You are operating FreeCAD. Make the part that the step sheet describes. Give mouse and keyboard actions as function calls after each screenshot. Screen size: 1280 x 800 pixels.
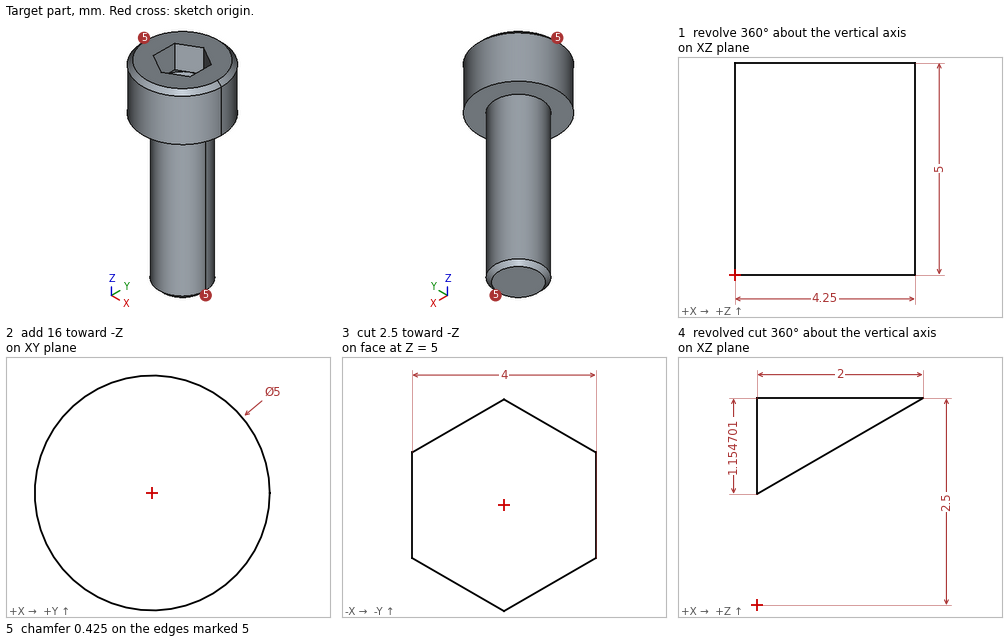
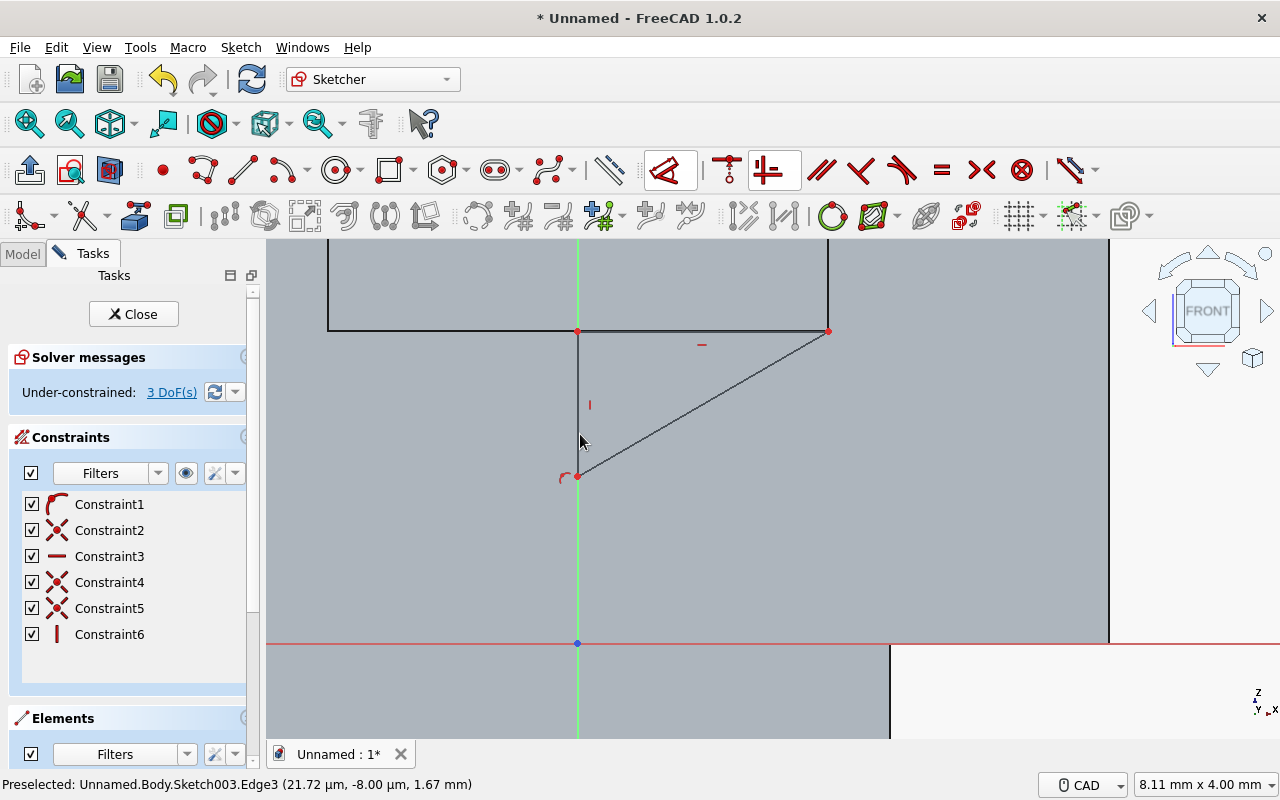
click(753, 332)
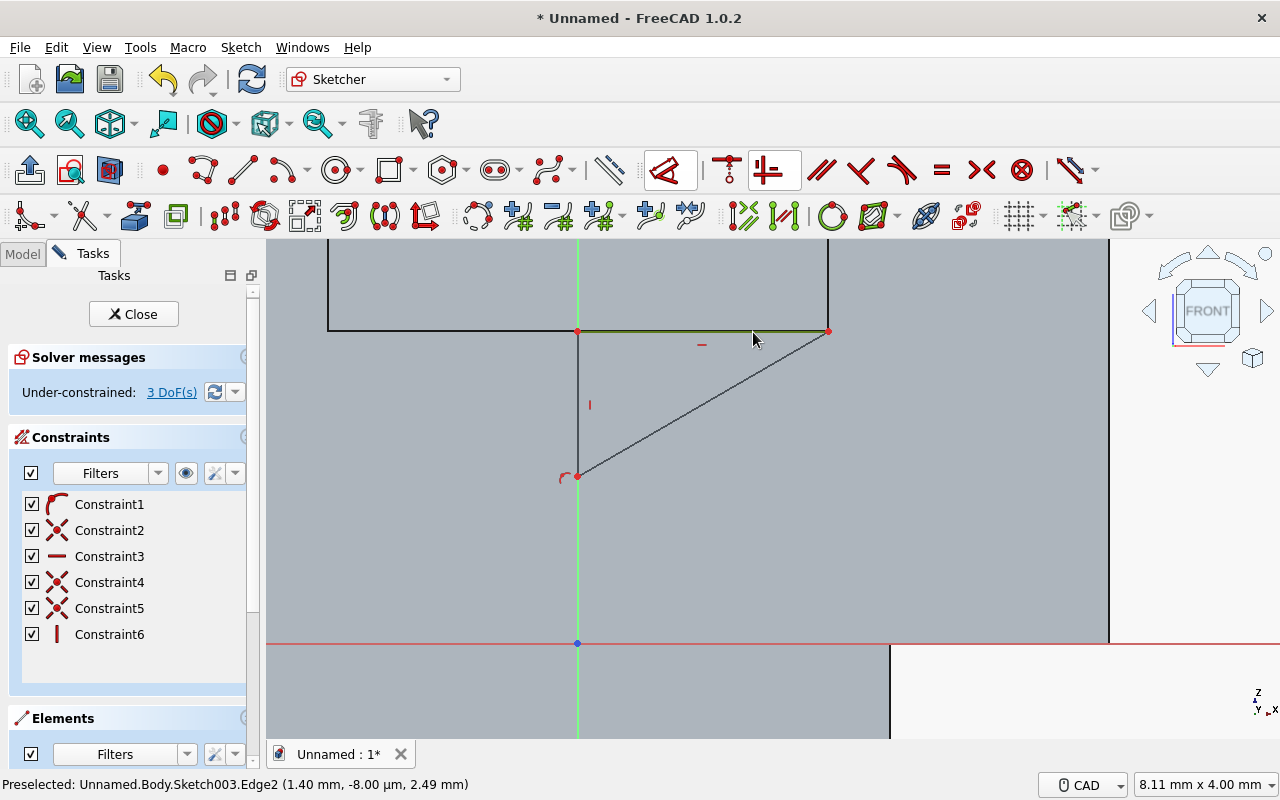
click(692, 170)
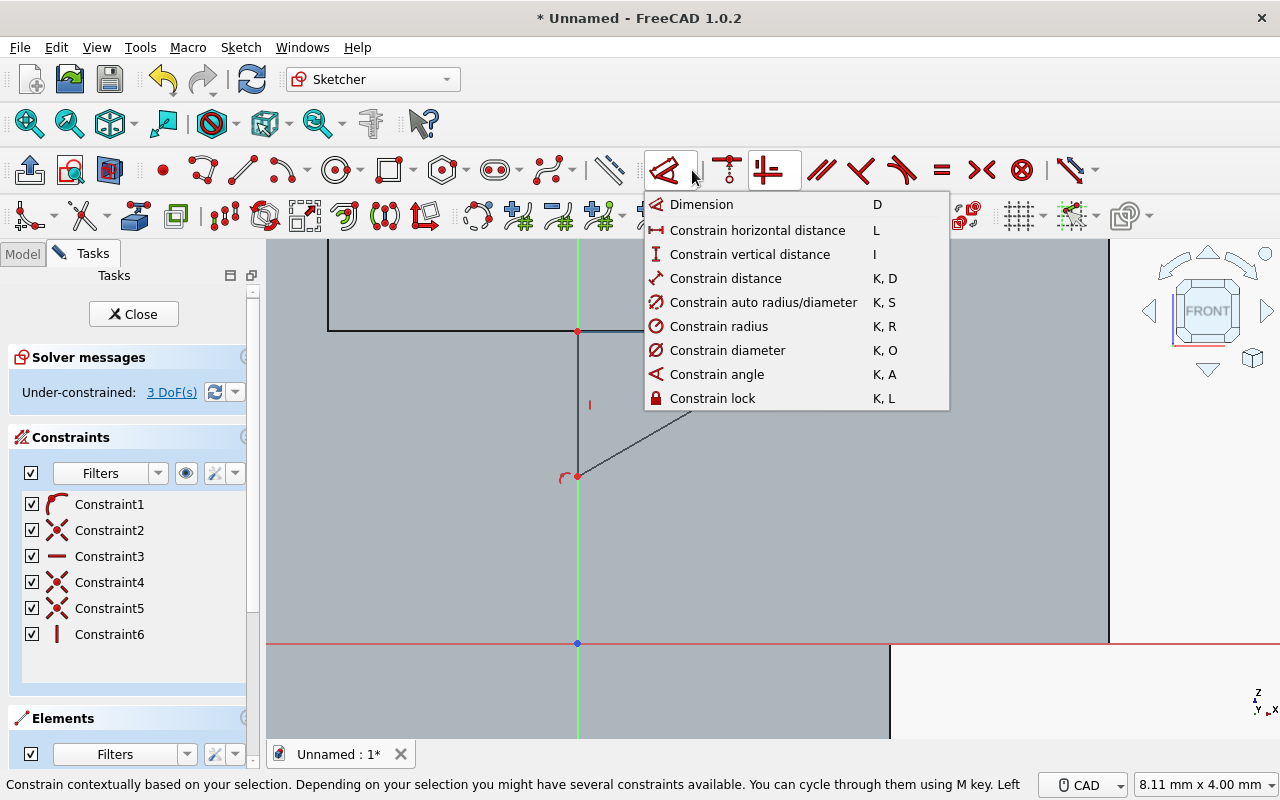
click(797, 230)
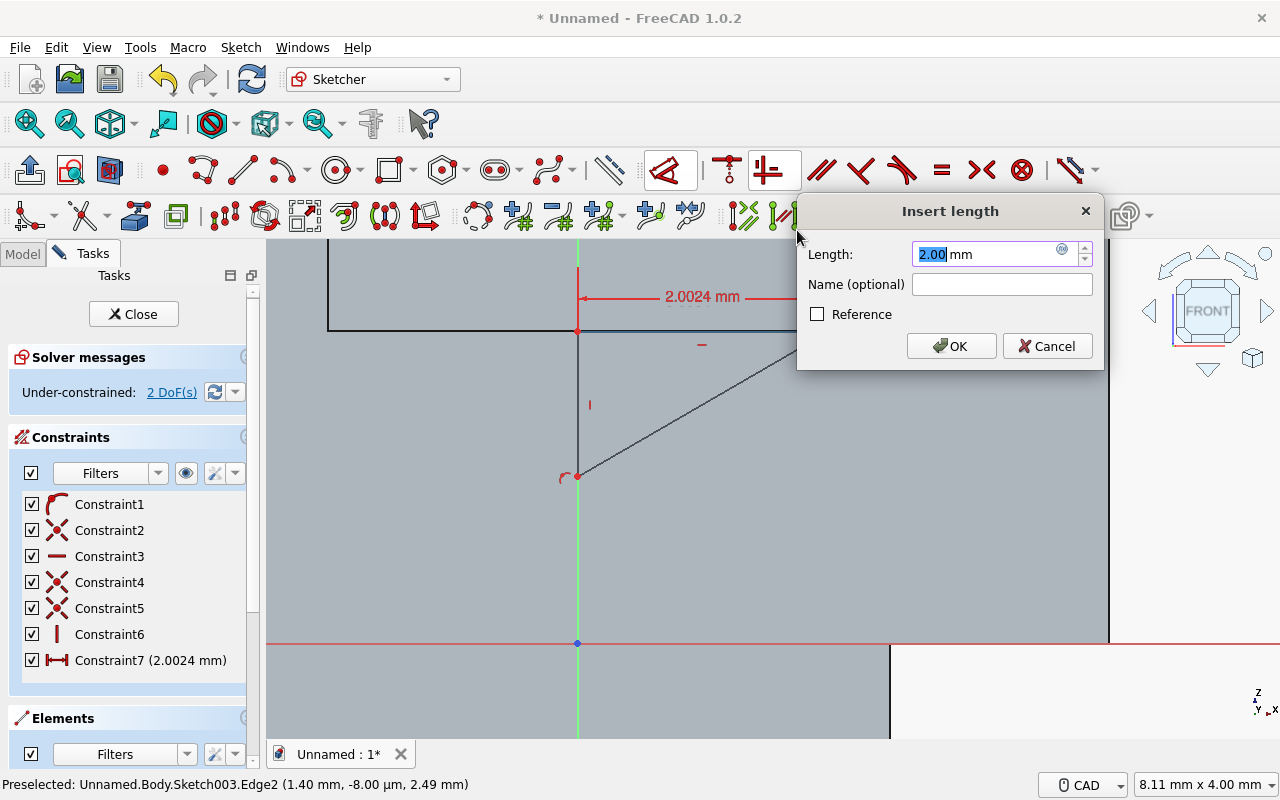
text(2)
key(Return)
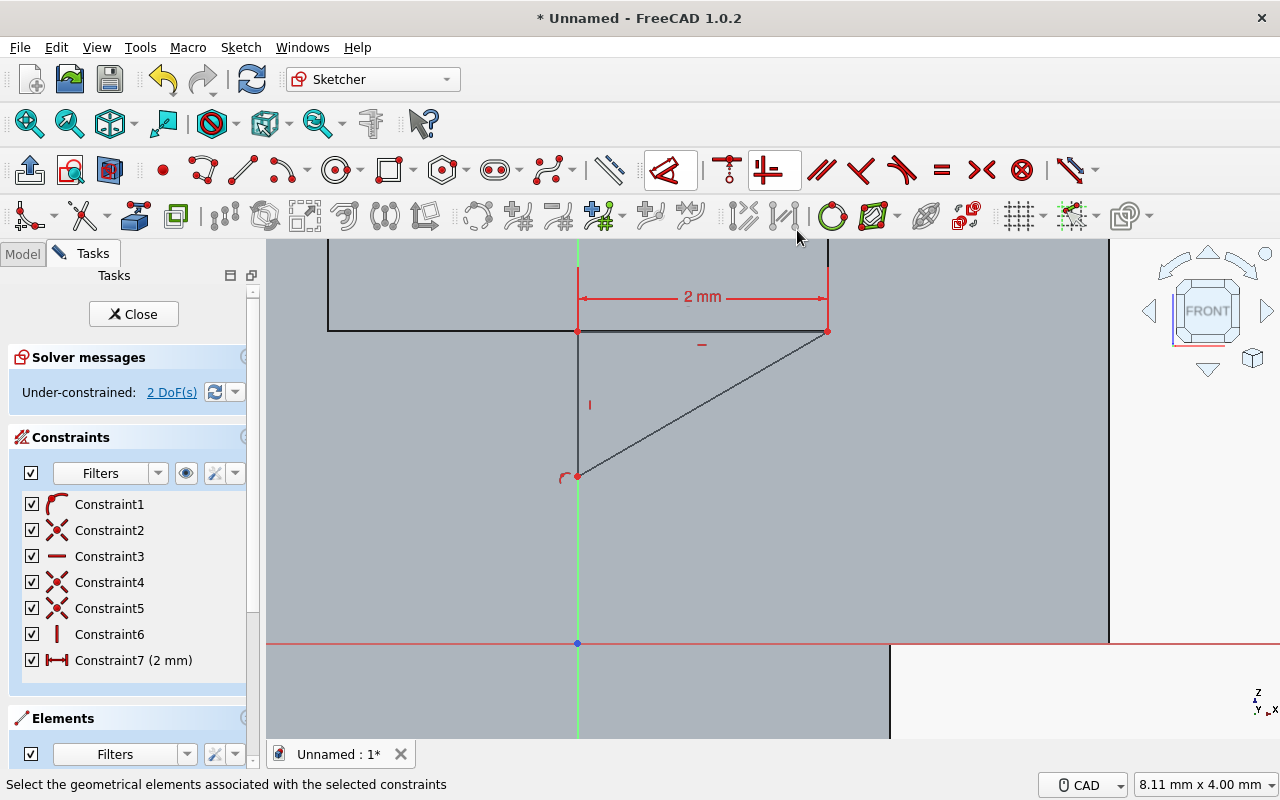
click(828, 332)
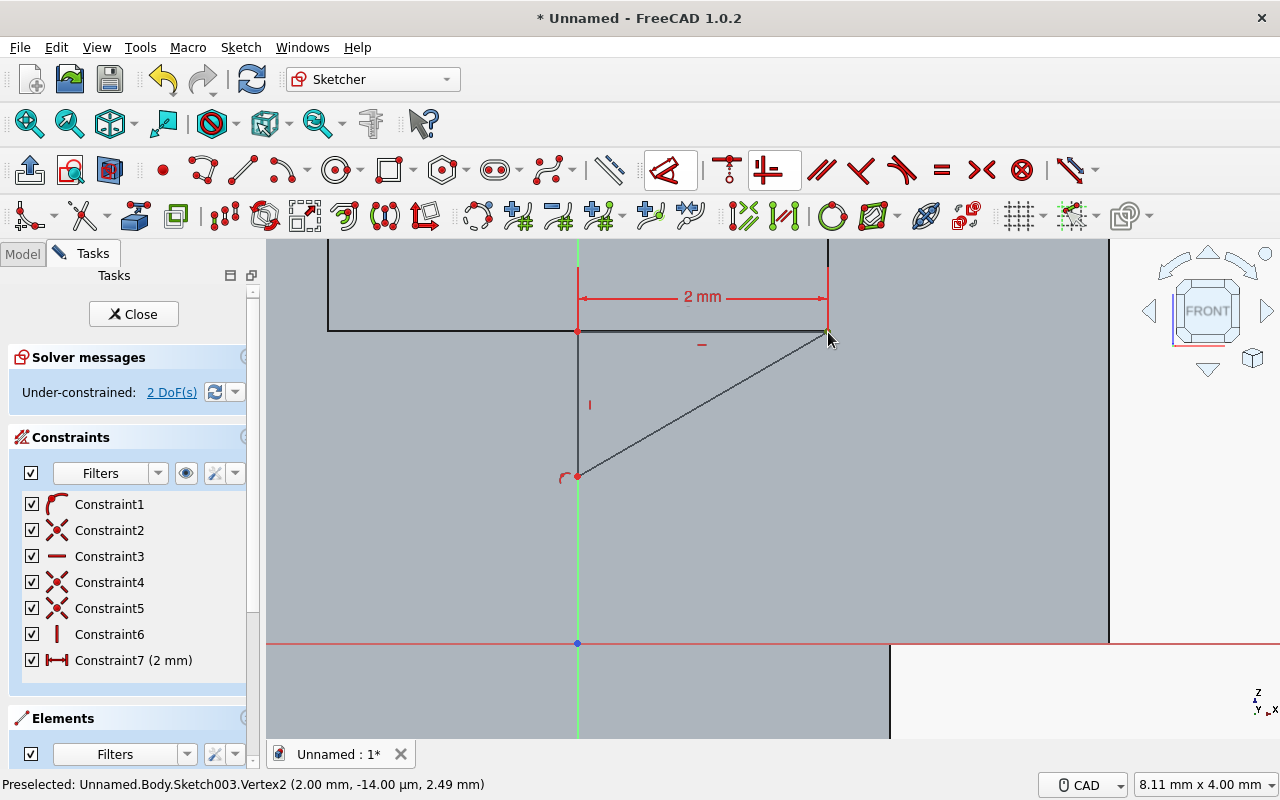
click(692, 170)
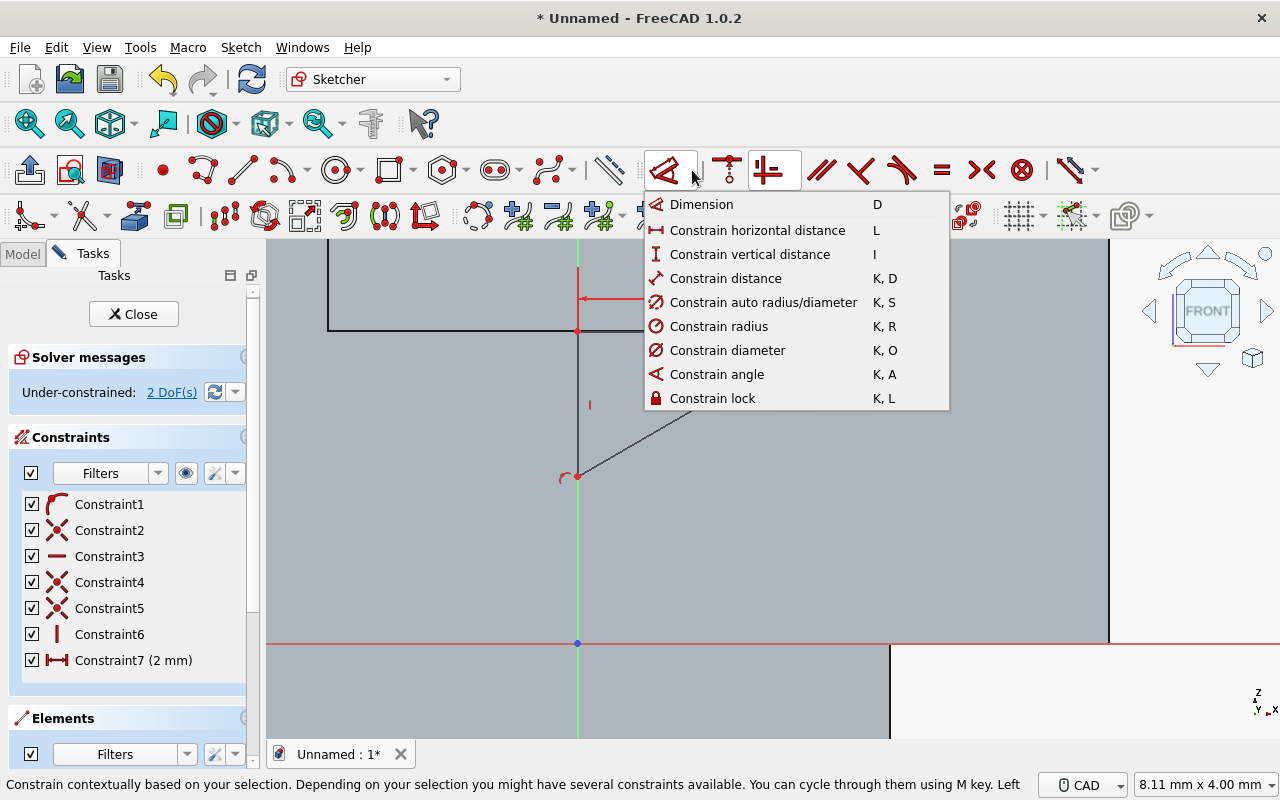
click(797, 254)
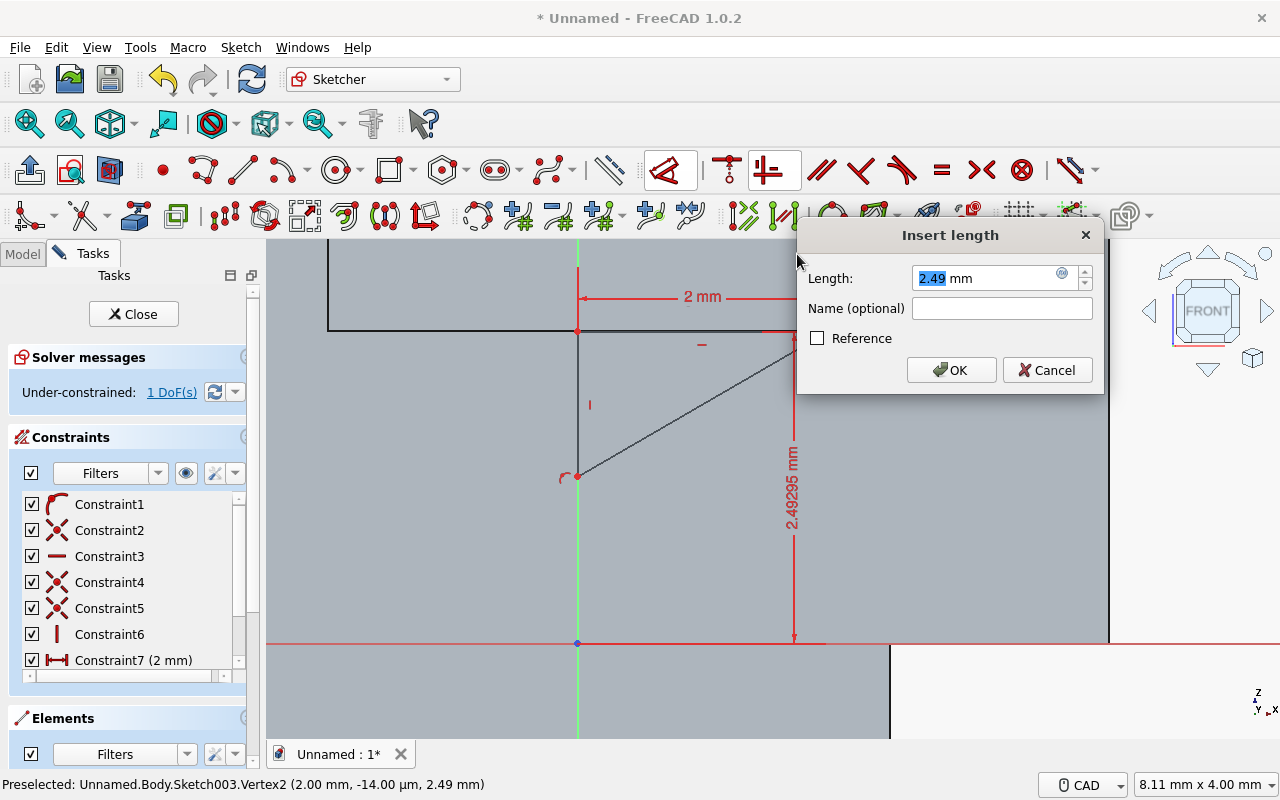
text(2.5)
key(Return)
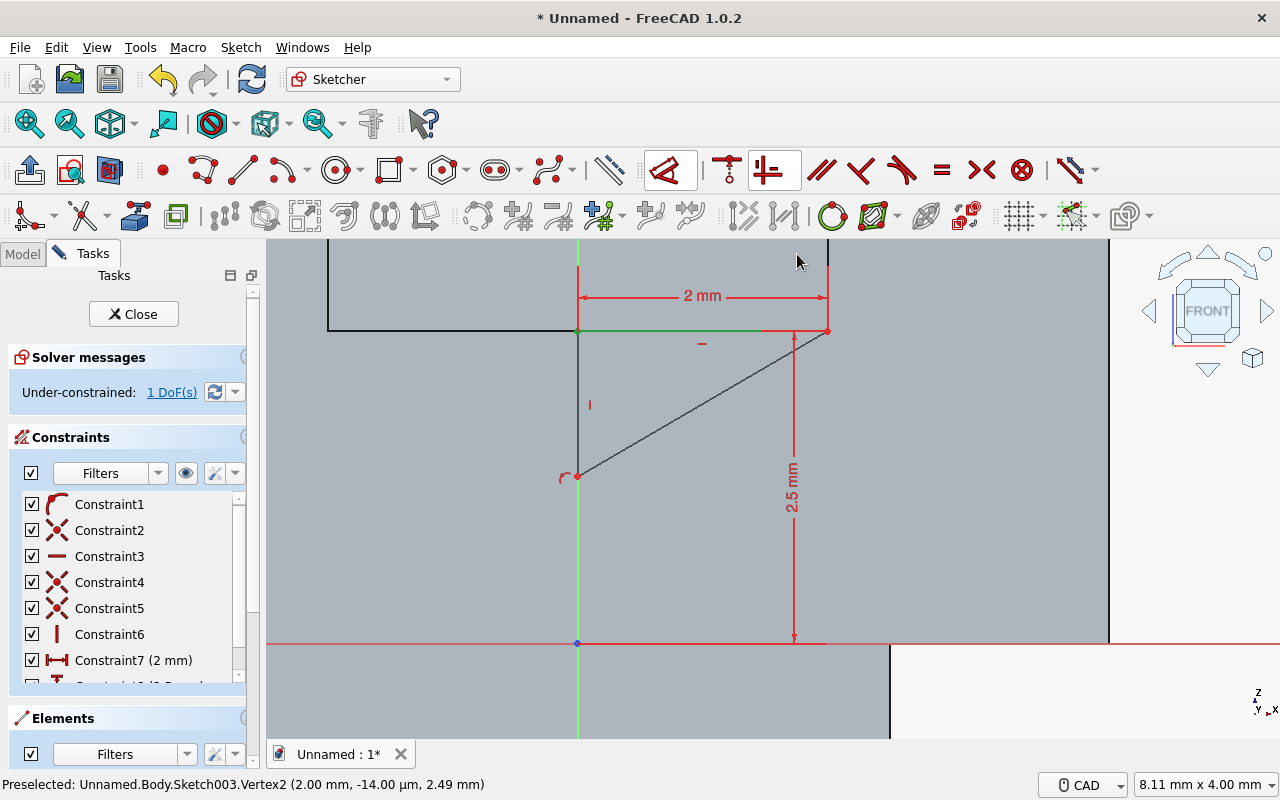
click(578, 375)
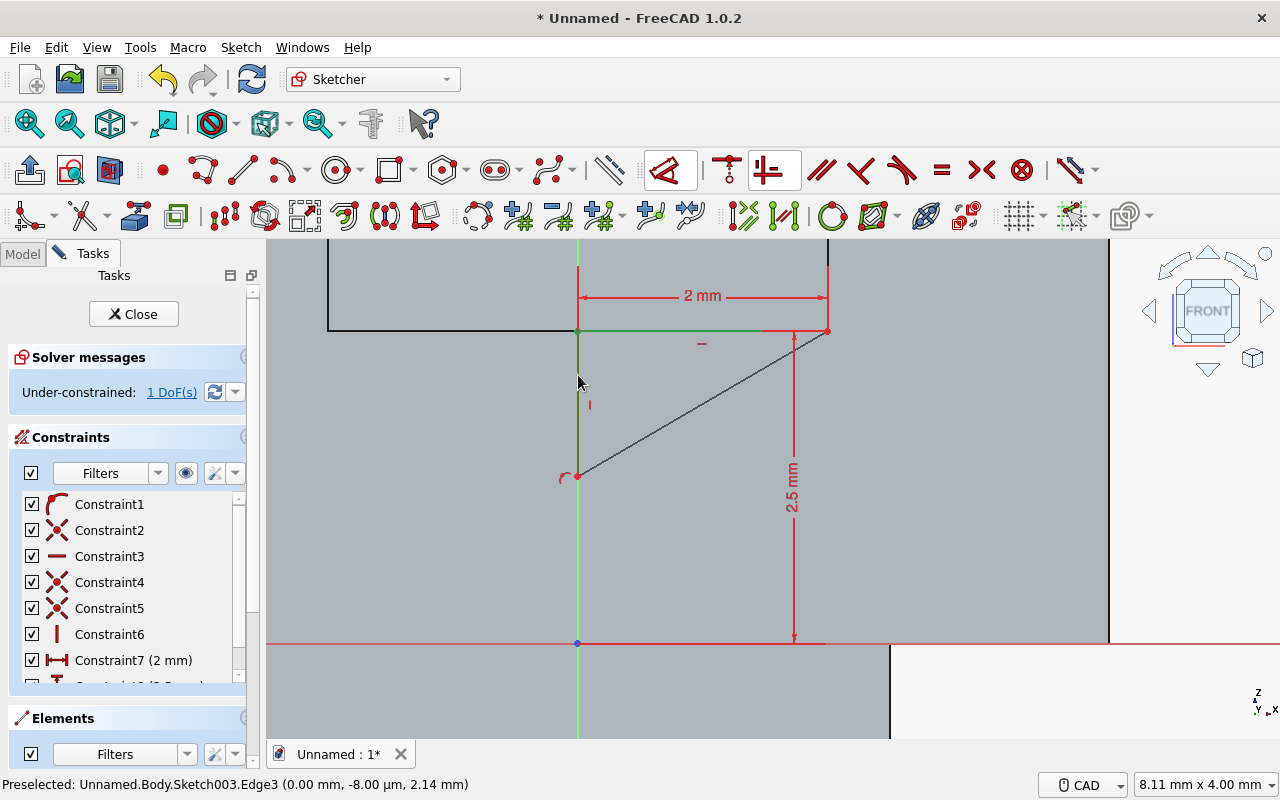
click(692, 170)